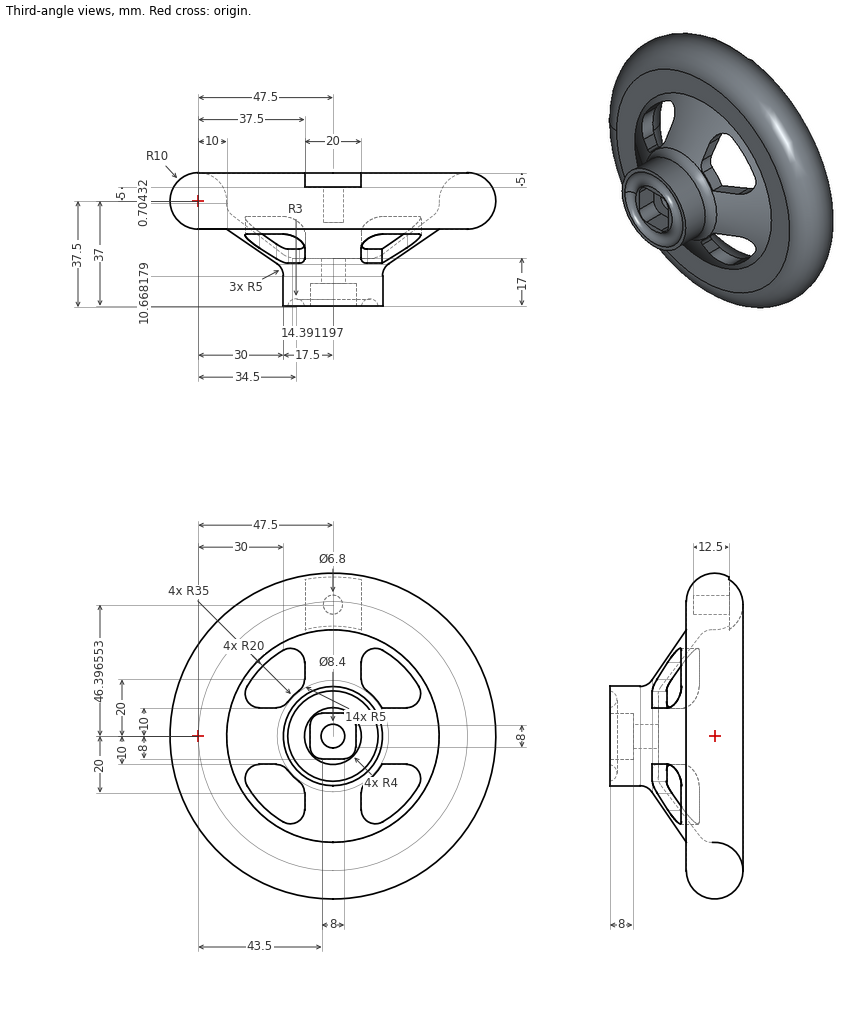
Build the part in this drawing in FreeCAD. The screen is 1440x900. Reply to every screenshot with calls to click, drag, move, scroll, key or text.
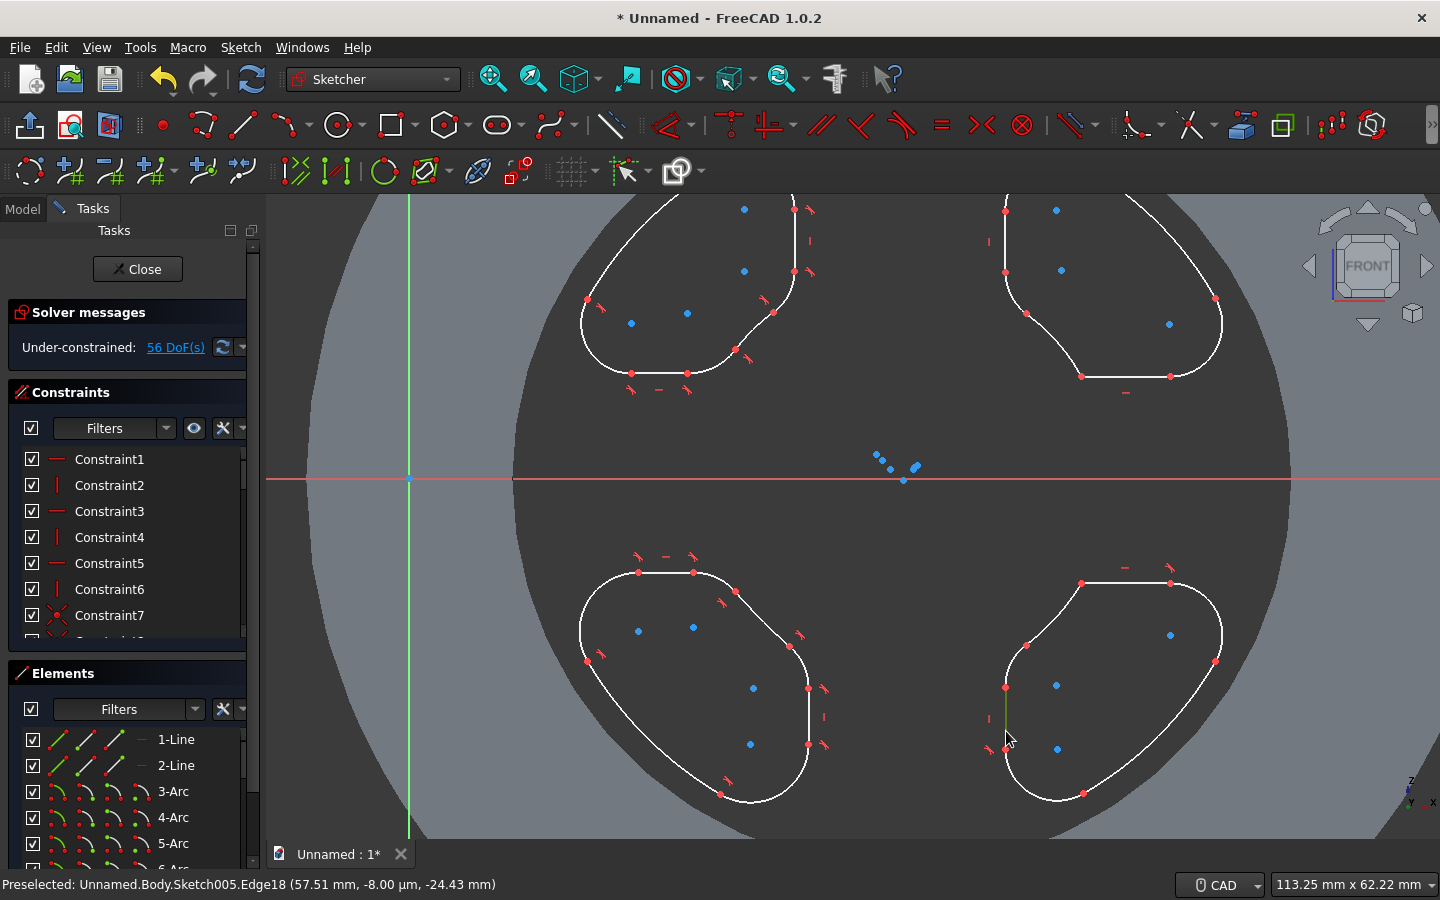
click(1016, 655)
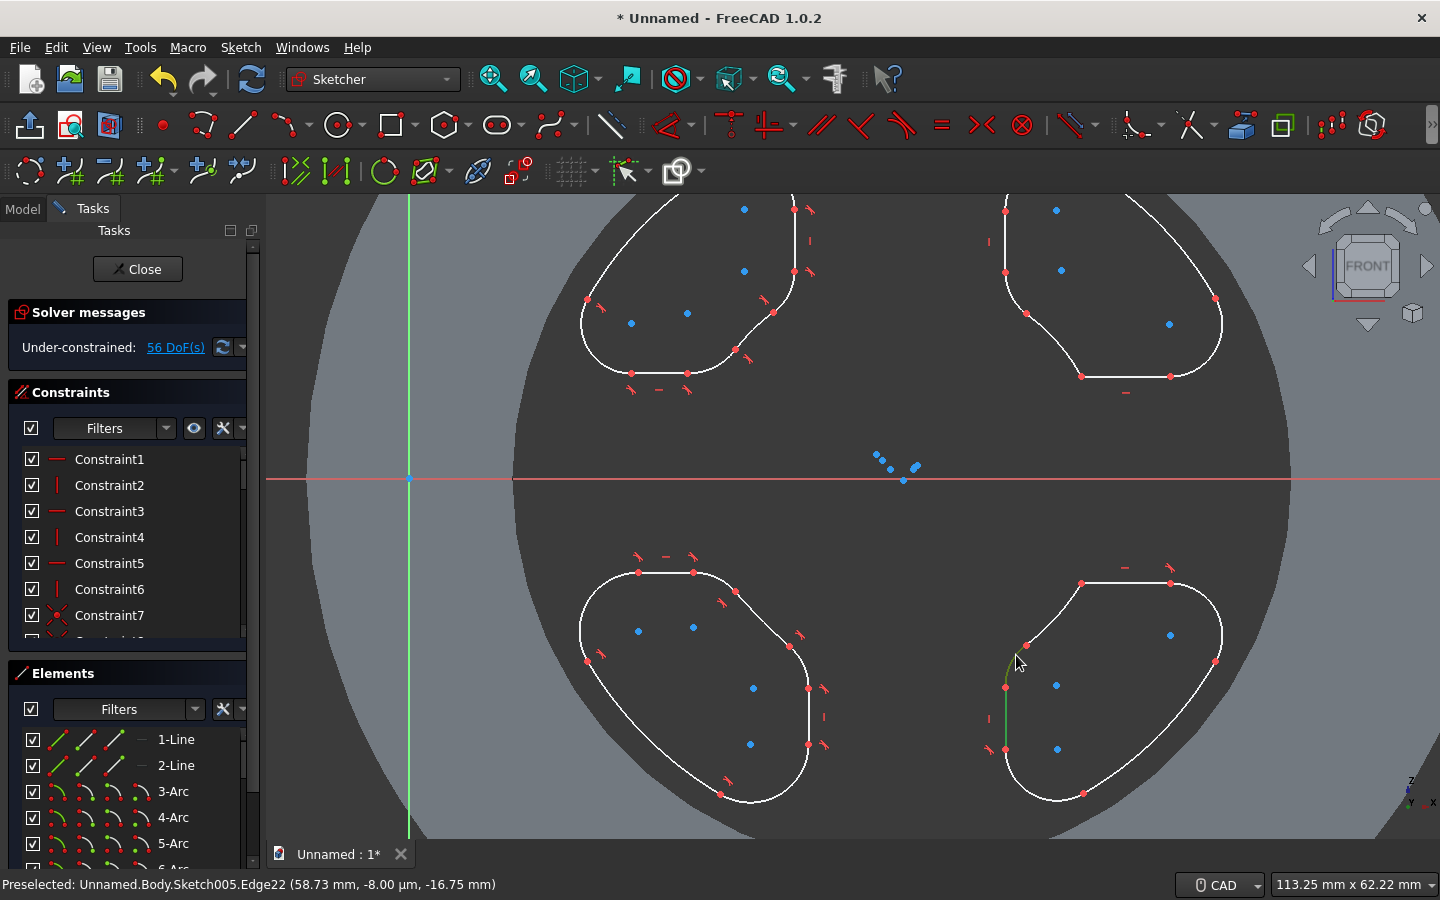
click(902, 126)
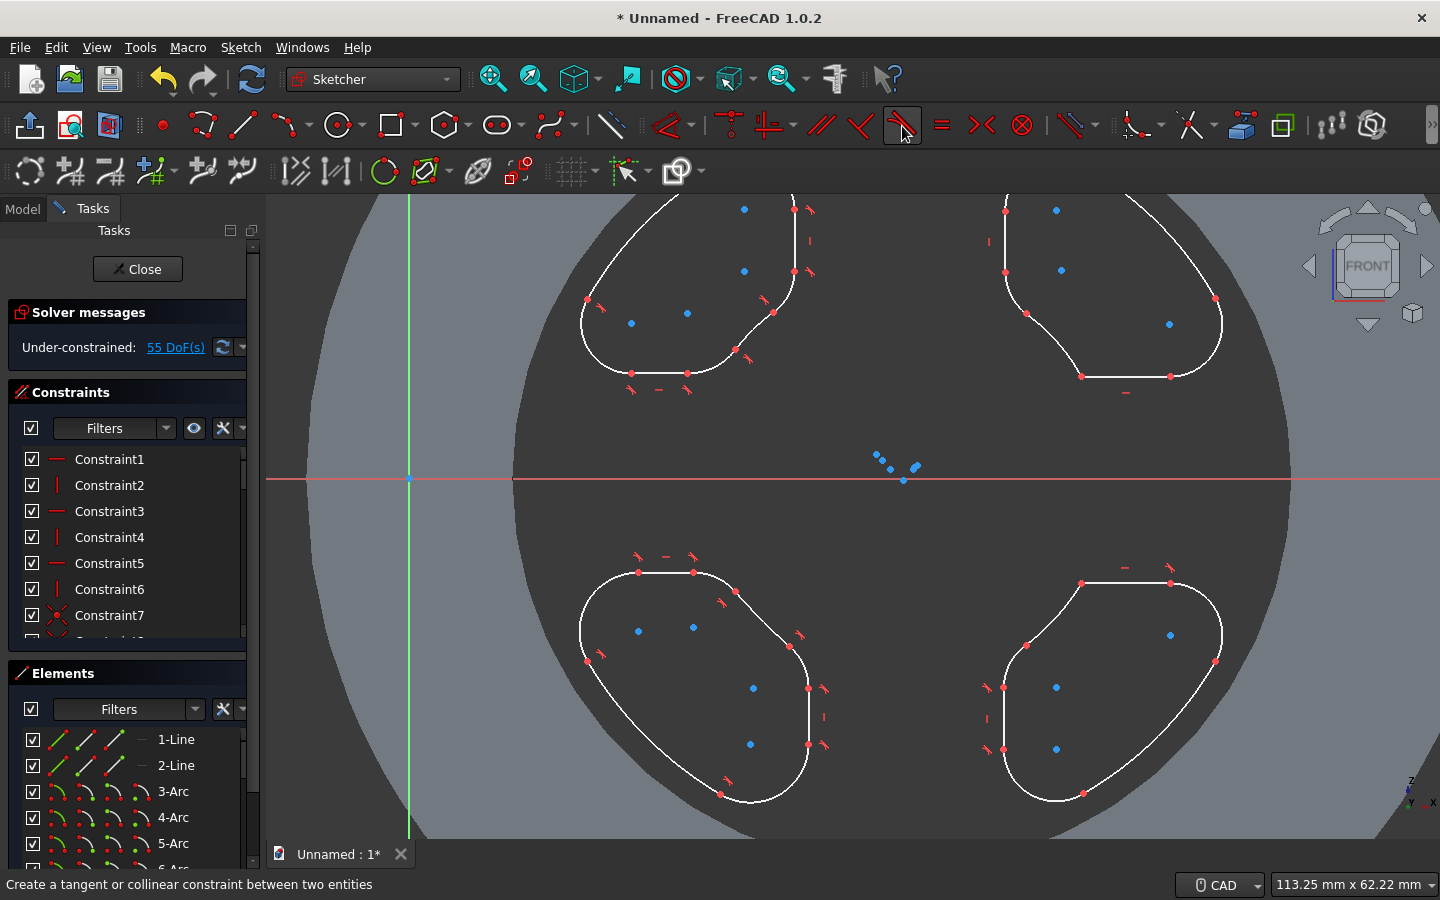
click(1222, 630)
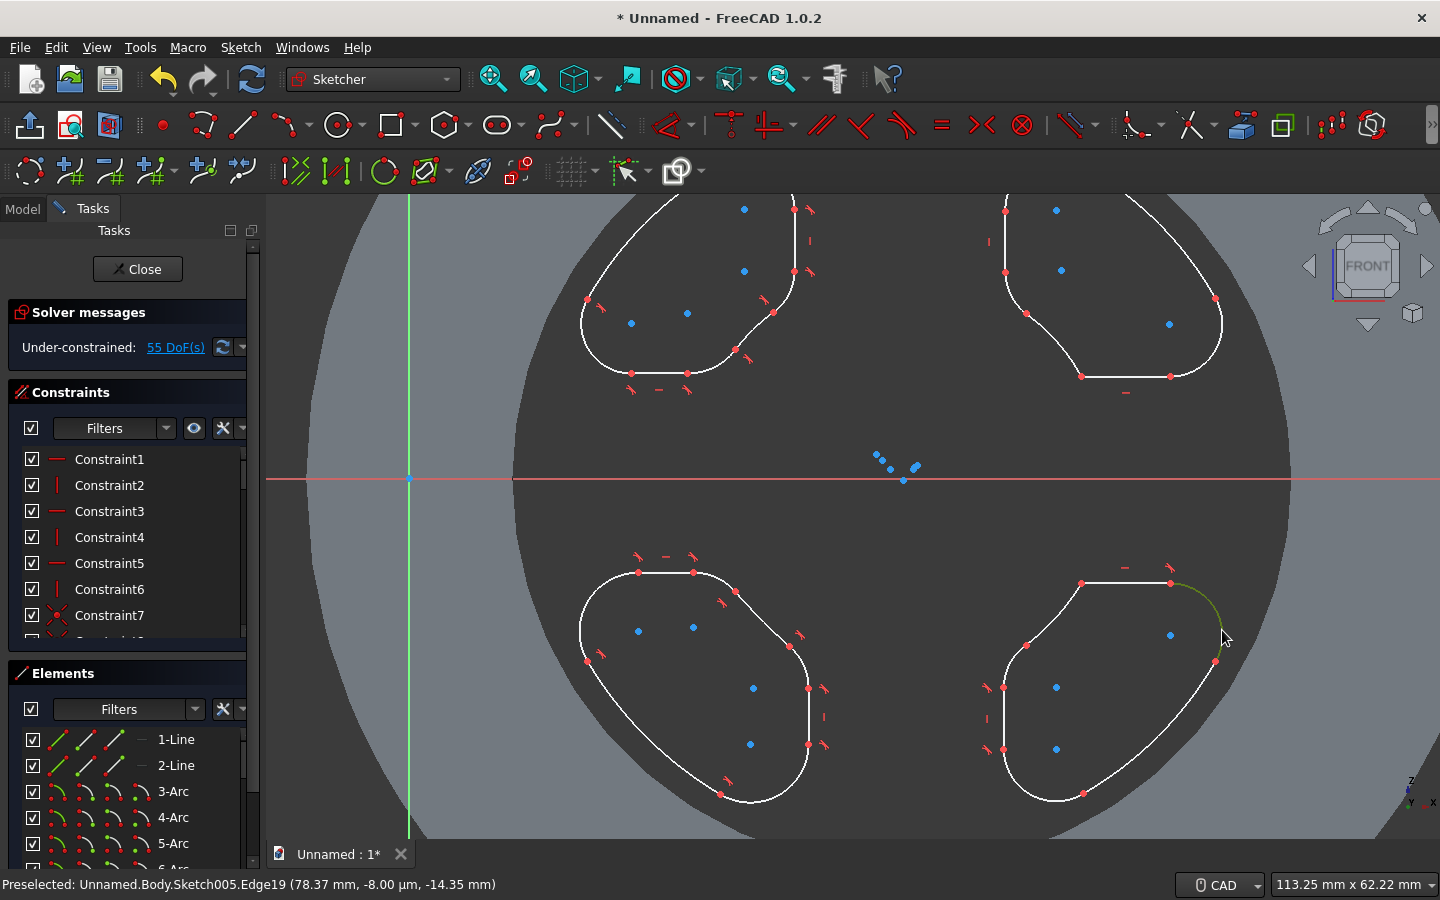
click(1130, 762)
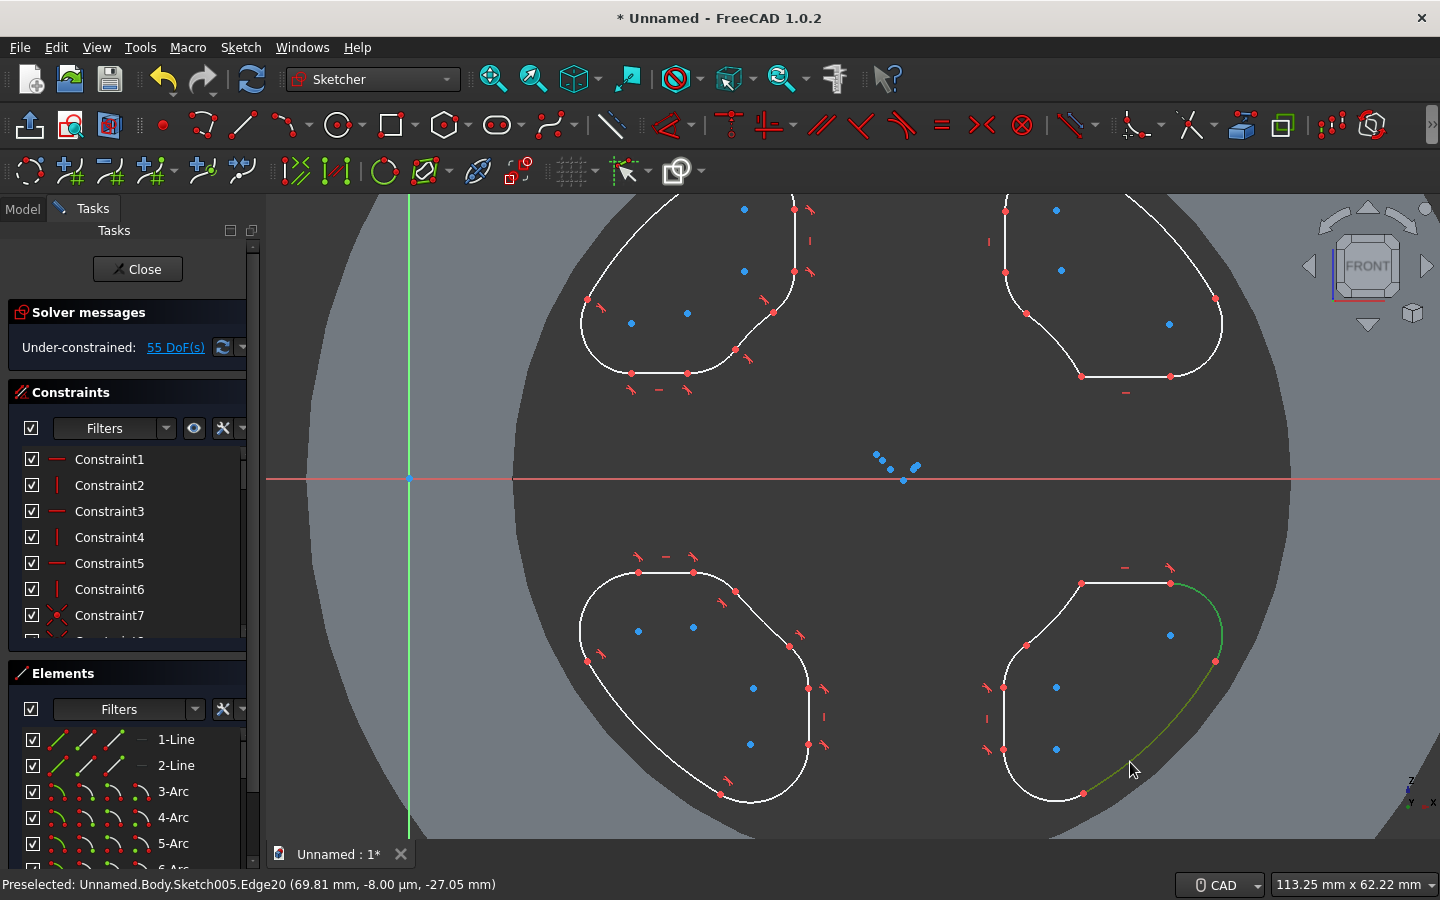
click(902, 126)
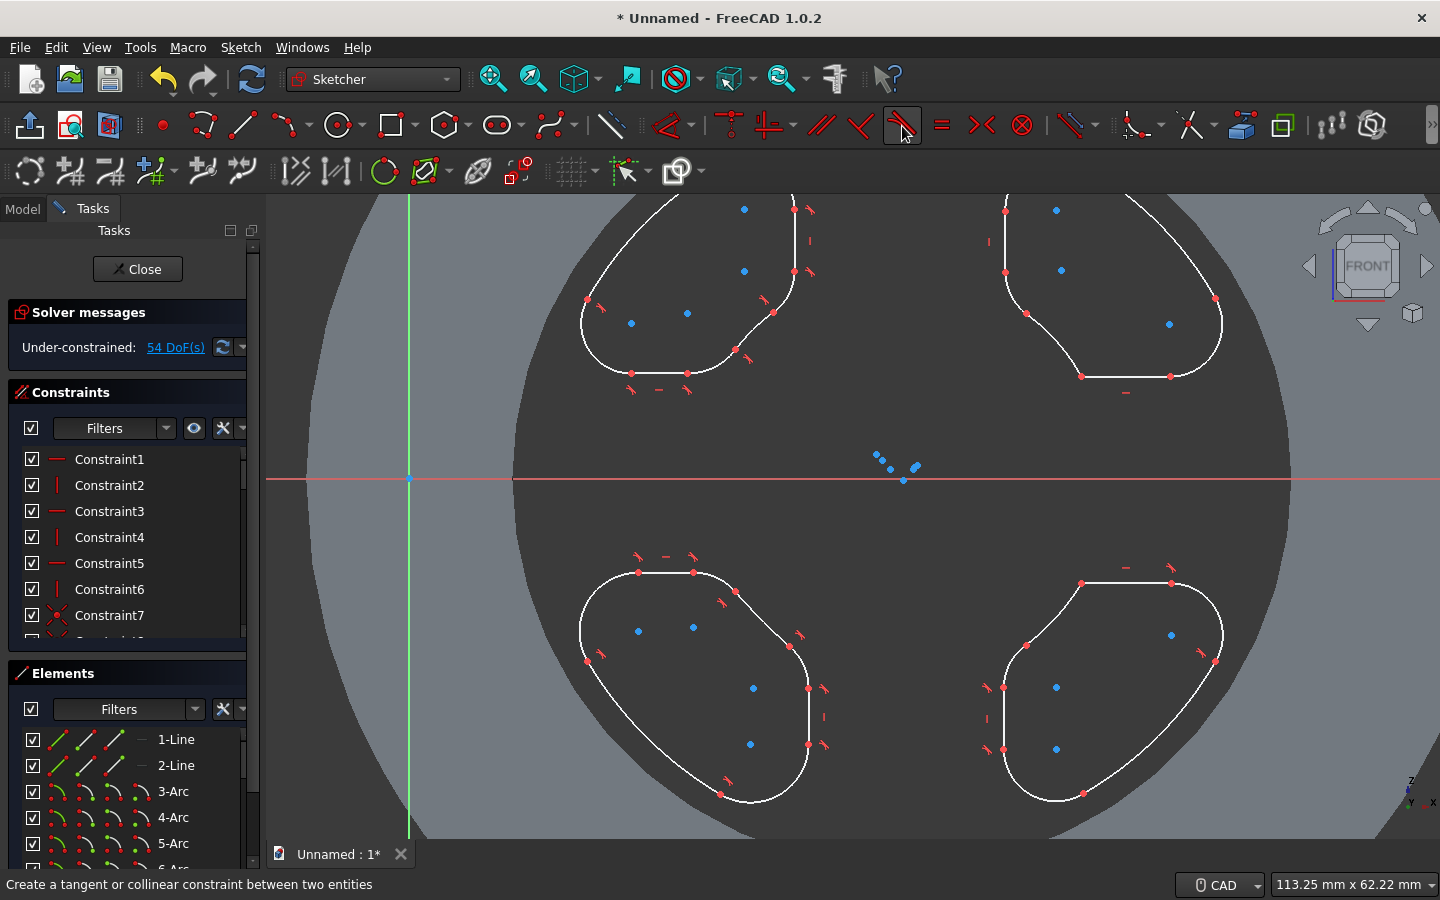
click(1130, 762)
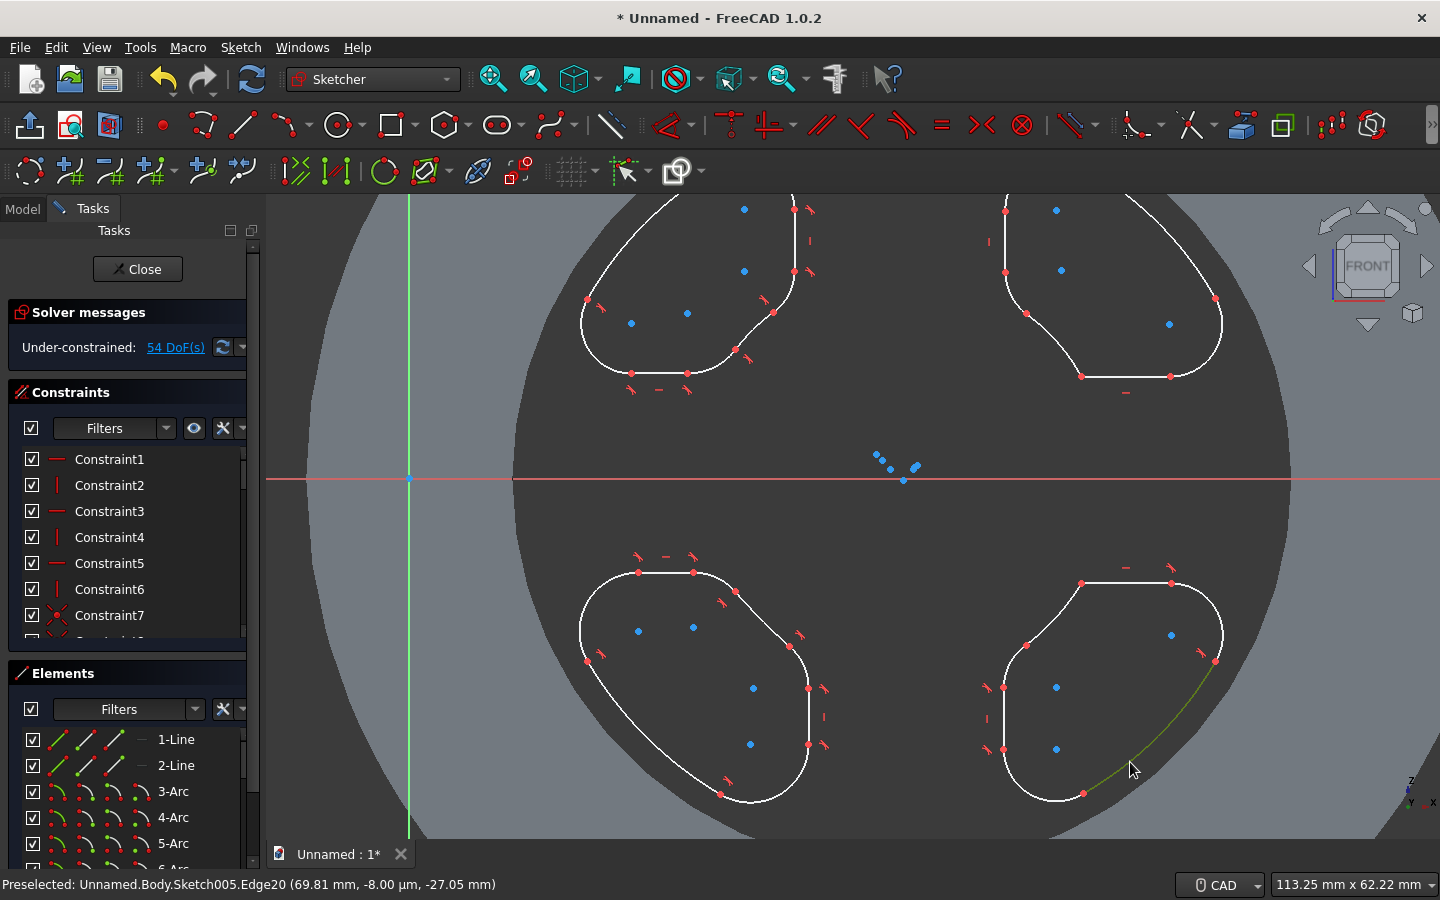
click(1014, 780)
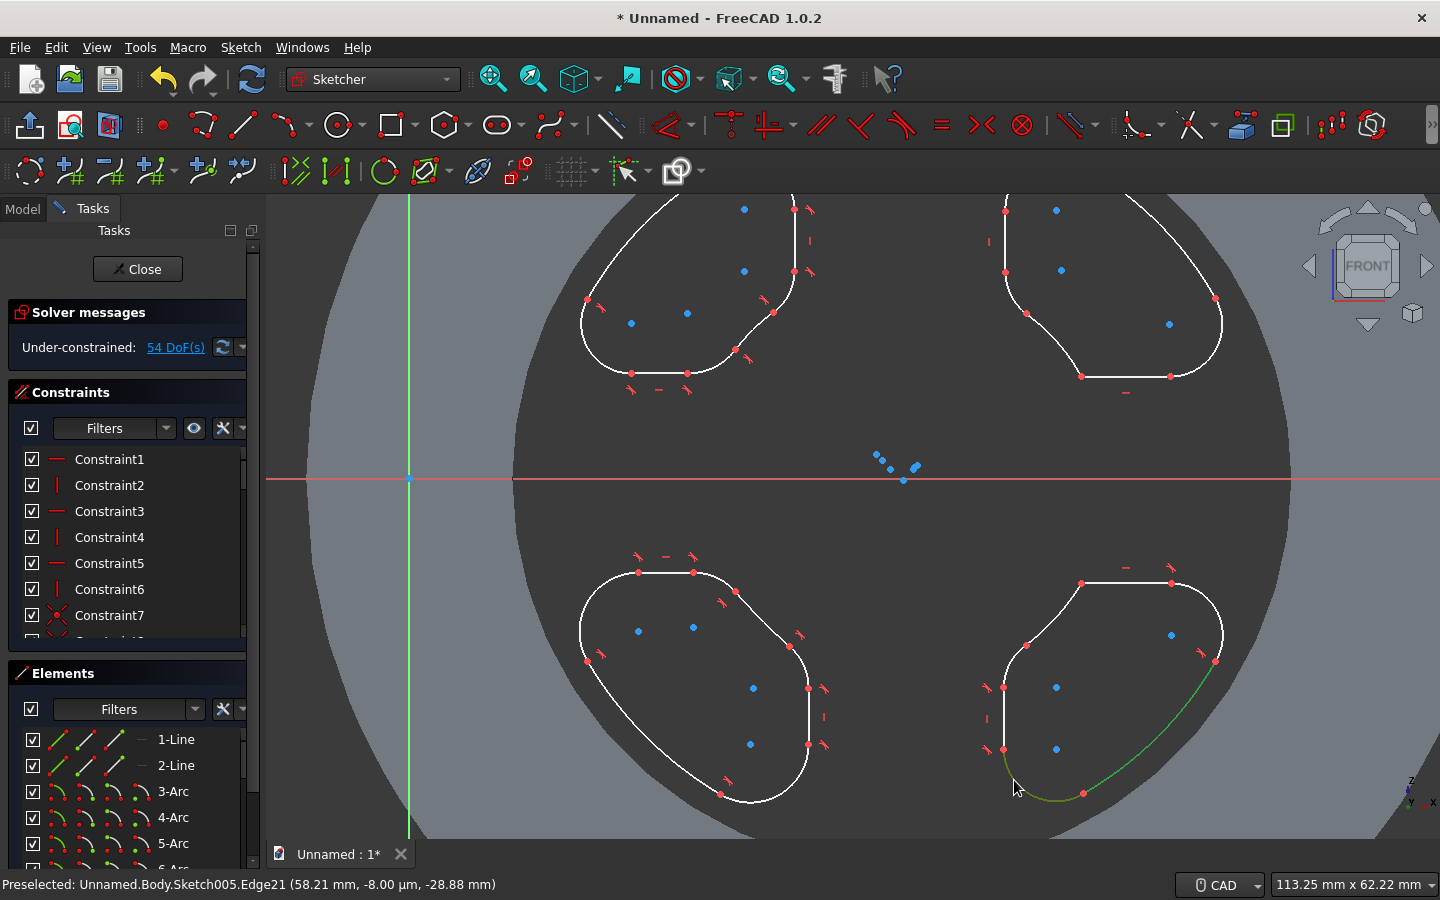
click(902, 126)